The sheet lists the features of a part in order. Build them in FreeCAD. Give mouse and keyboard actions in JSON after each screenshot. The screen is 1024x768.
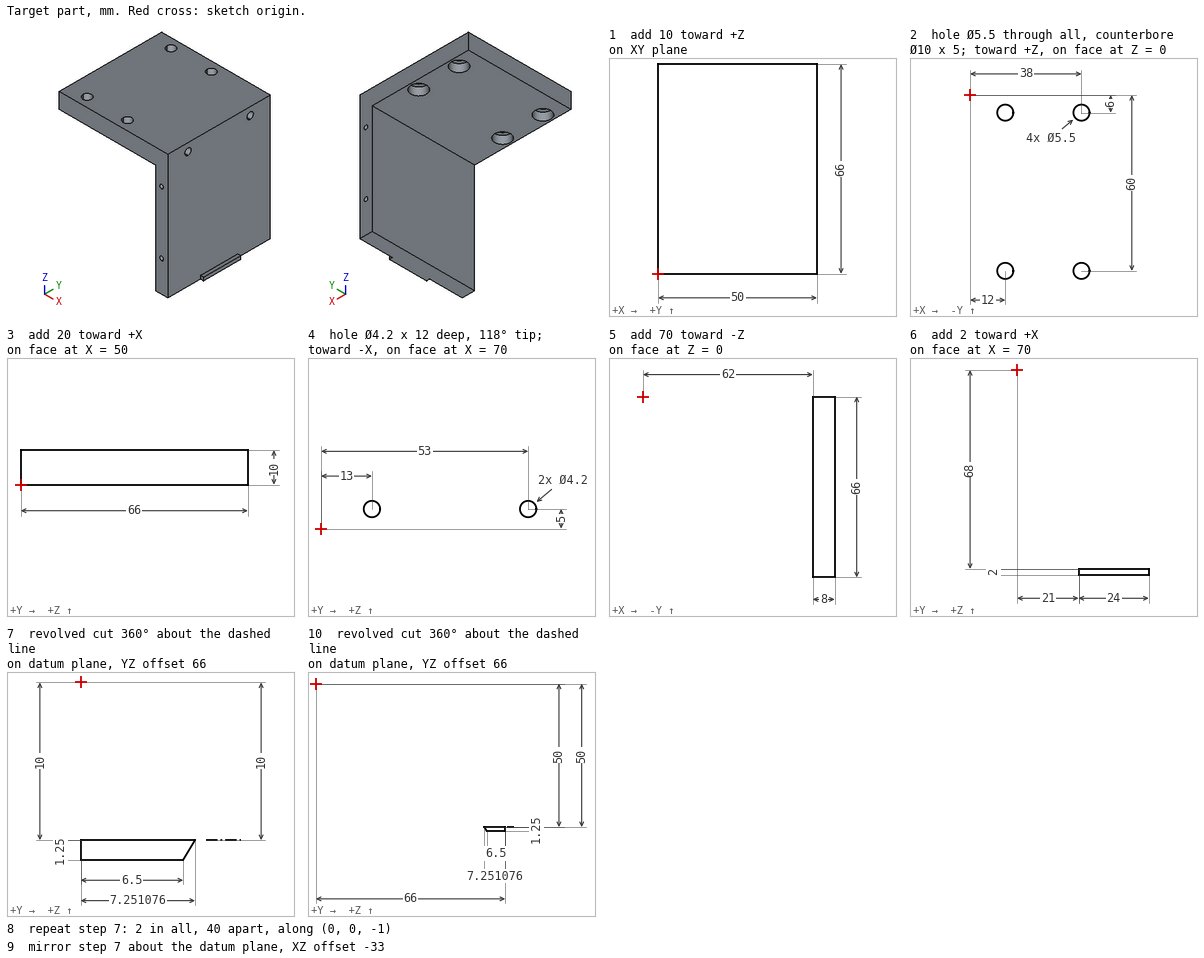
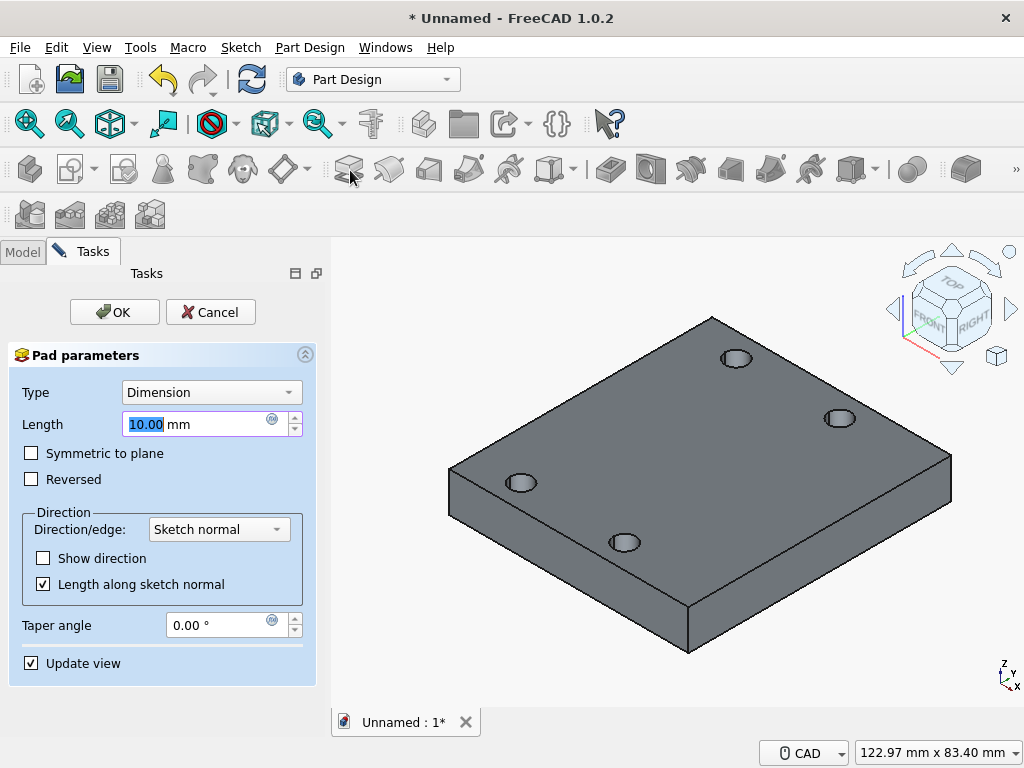
{"action": "type", "text": "20"}
{"action": "key", "text": "Tab"}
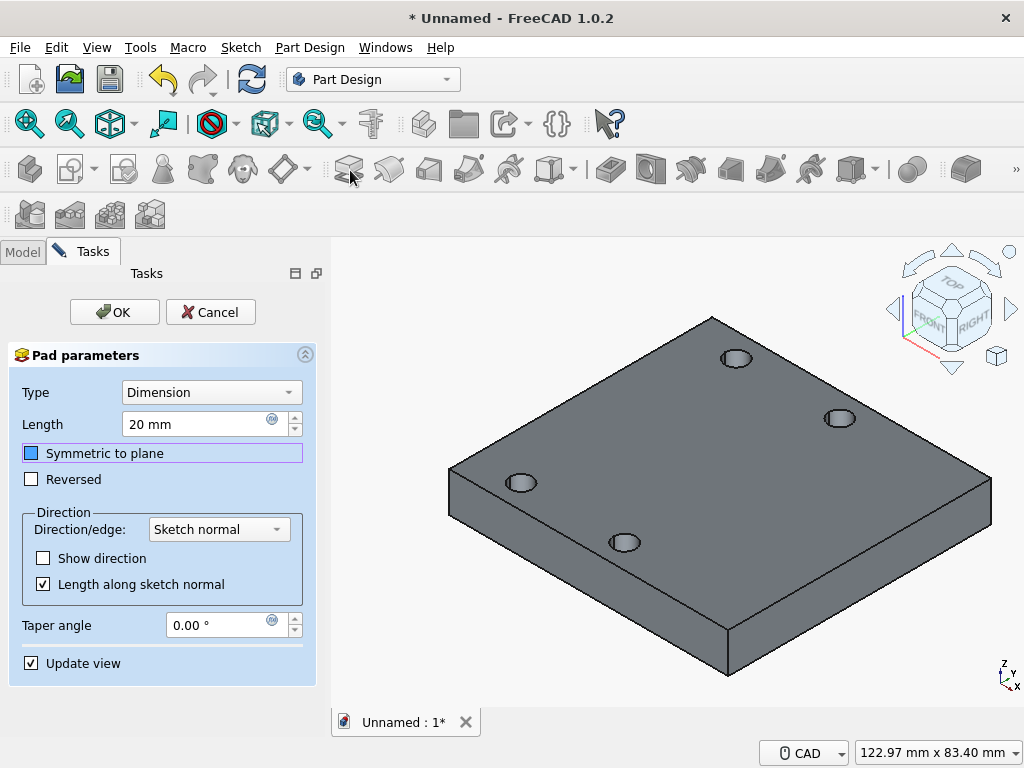
{"action": "left_click", "coordinate": [115, 312]}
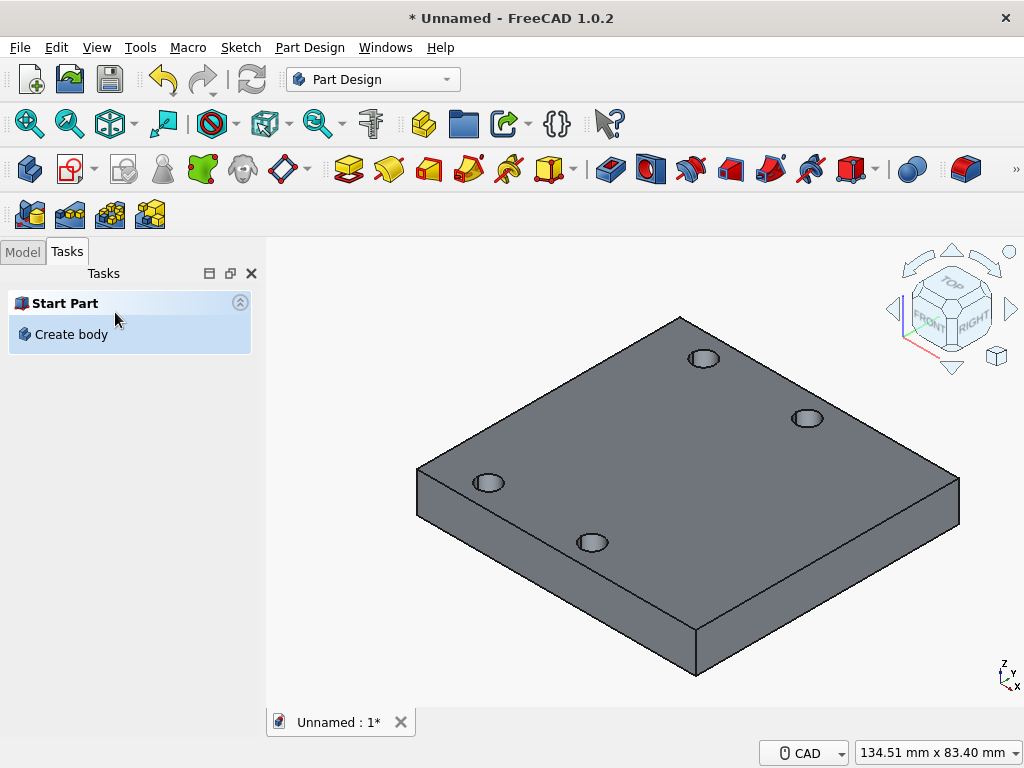
{"action": "left_click", "coordinate": [902, 533]}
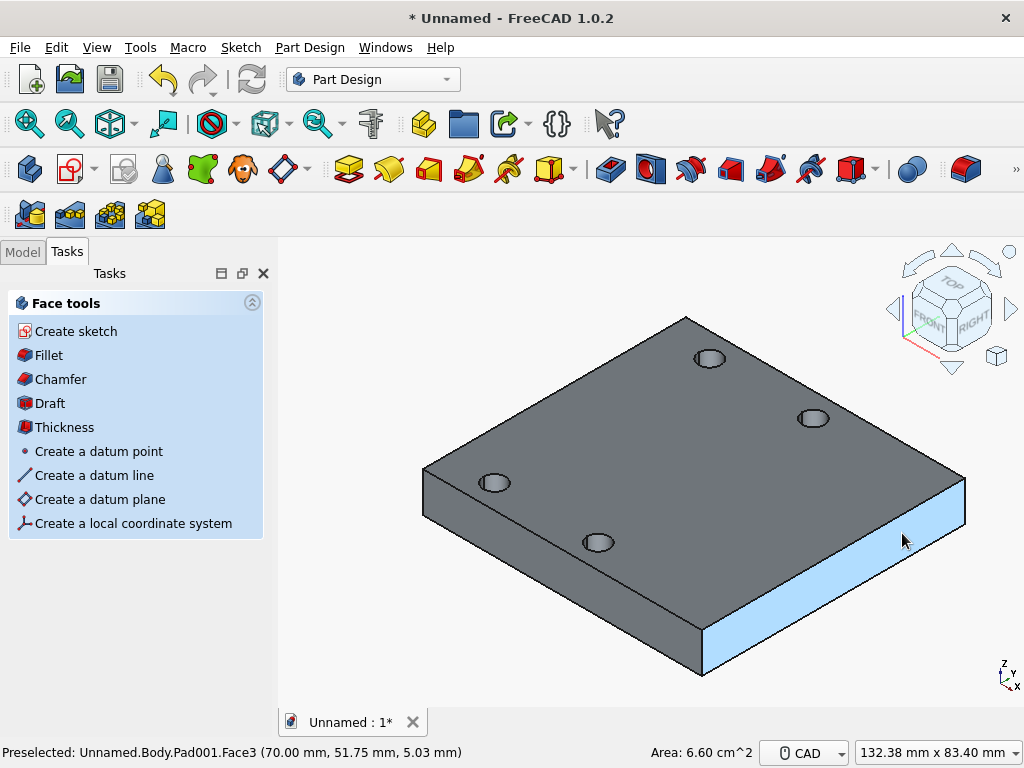
{"action": "left_click", "coordinate": [70, 170]}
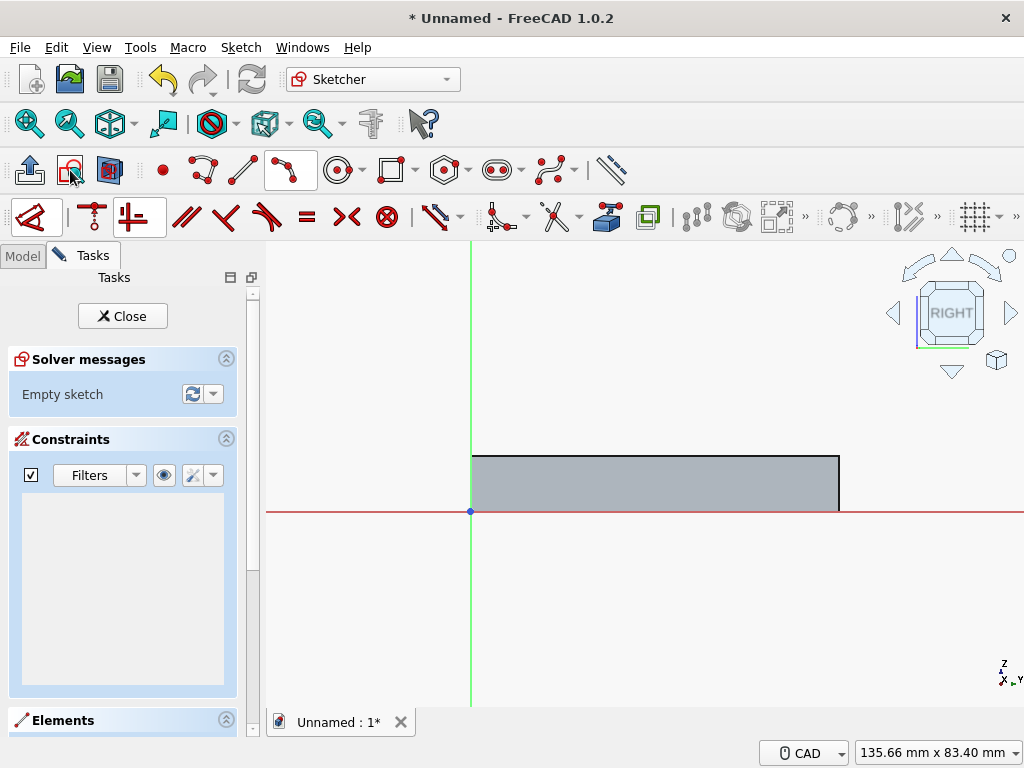
{"action": "key", "text": "g c"}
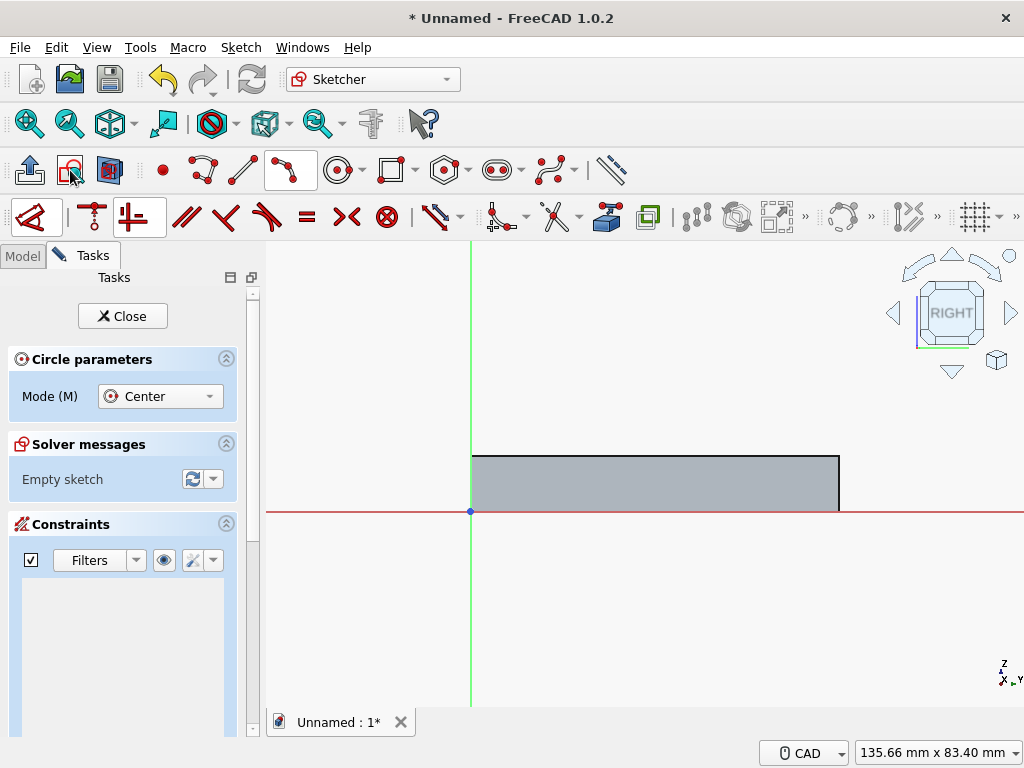
{"action": "scroll", "coordinate": [767, 484], "scroll_direction": "up", "scroll_amount": 4}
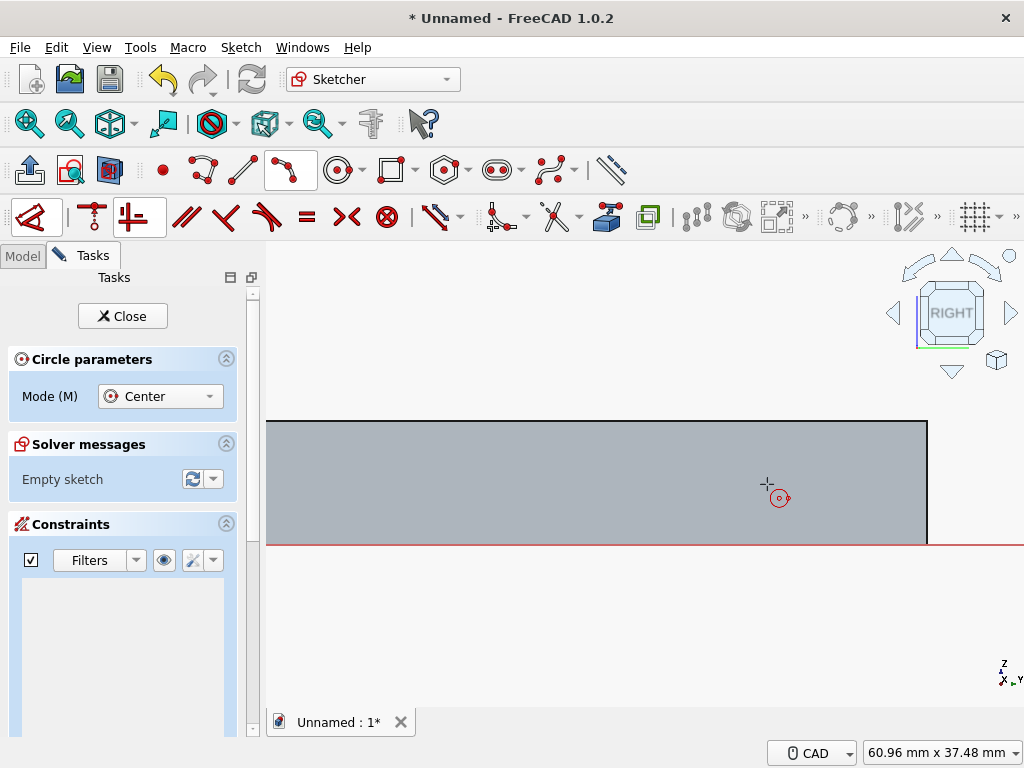
{"action": "left_click", "coordinate": [765, 483]}
{"action": "left_click", "coordinate": [784, 465]}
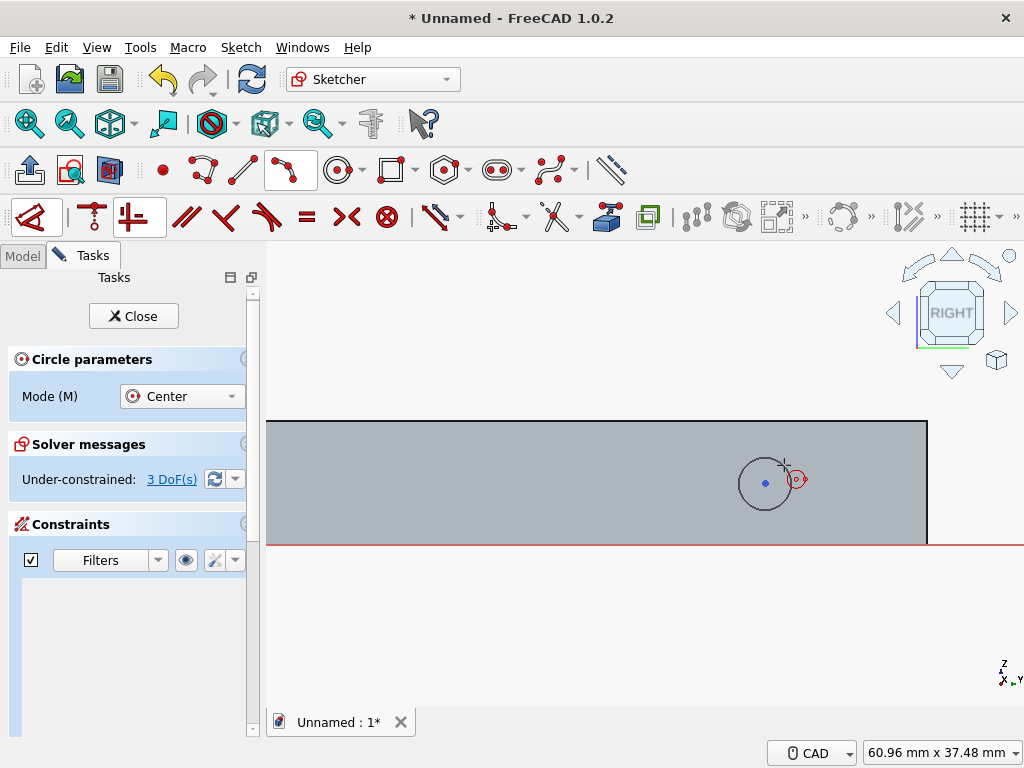
{"action": "scroll", "coordinate": [732, 441], "scroll_direction": "down", "scroll_amount": 3}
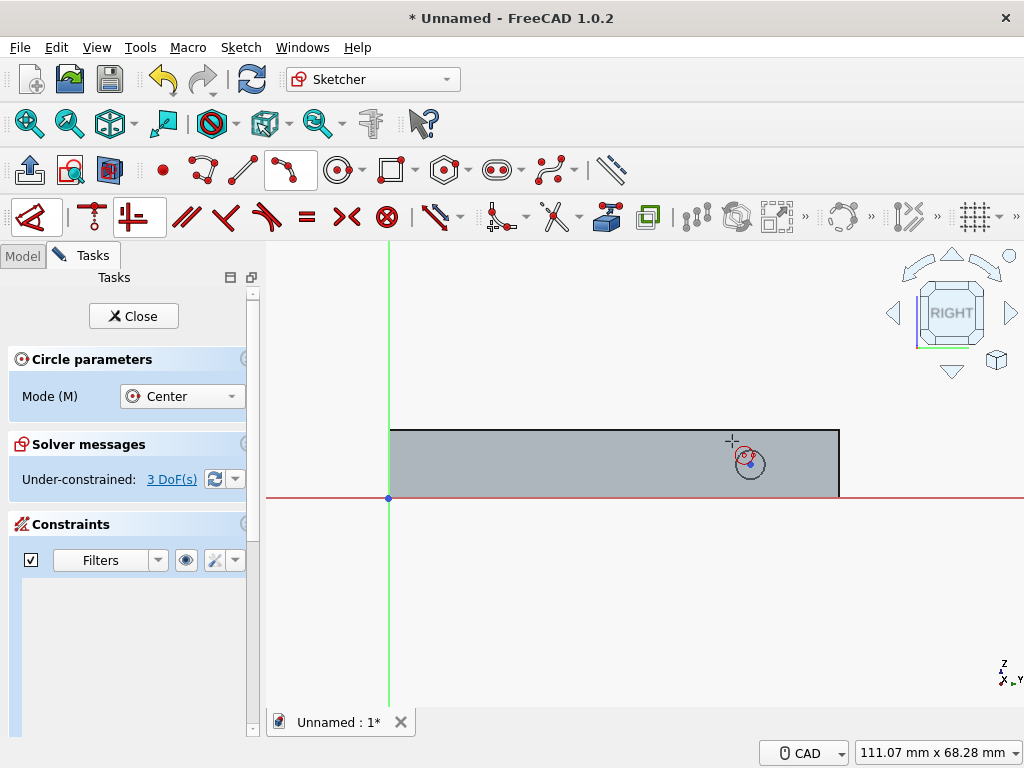
{"action": "scroll", "coordinate": [478, 464], "scroll_direction": "up", "scroll_amount": 3}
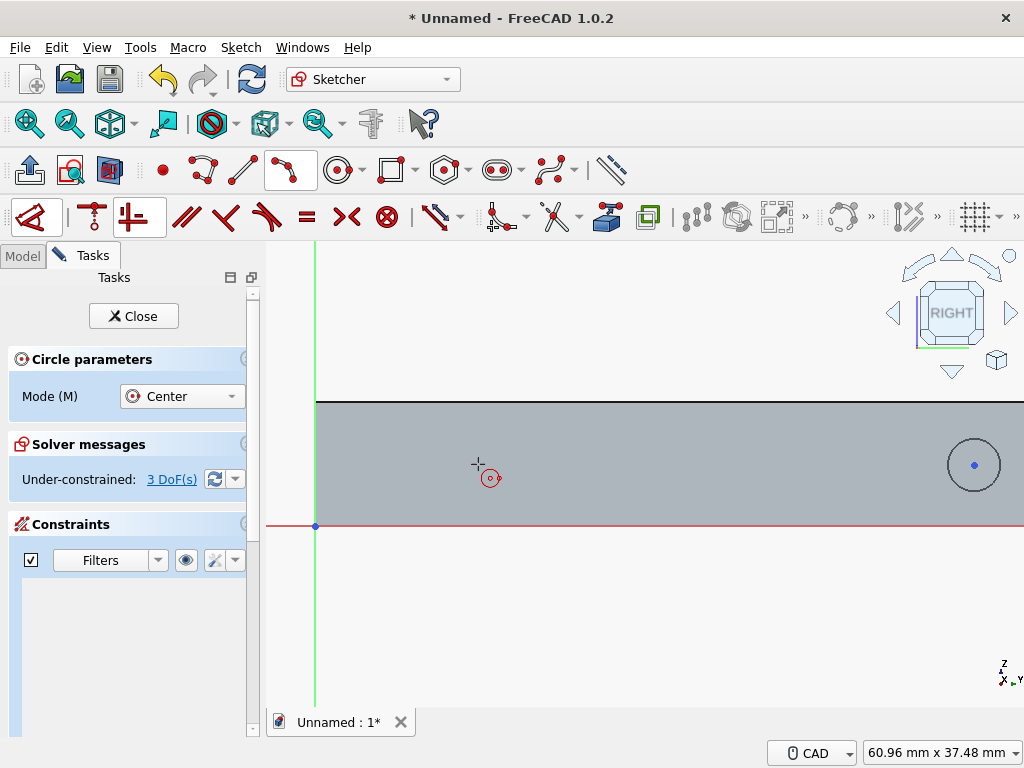
{"action": "left_click", "coordinate": [477, 464]}
{"action": "left_click", "coordinate": [496, 446]}
{"action": "key", "text": "Escape"}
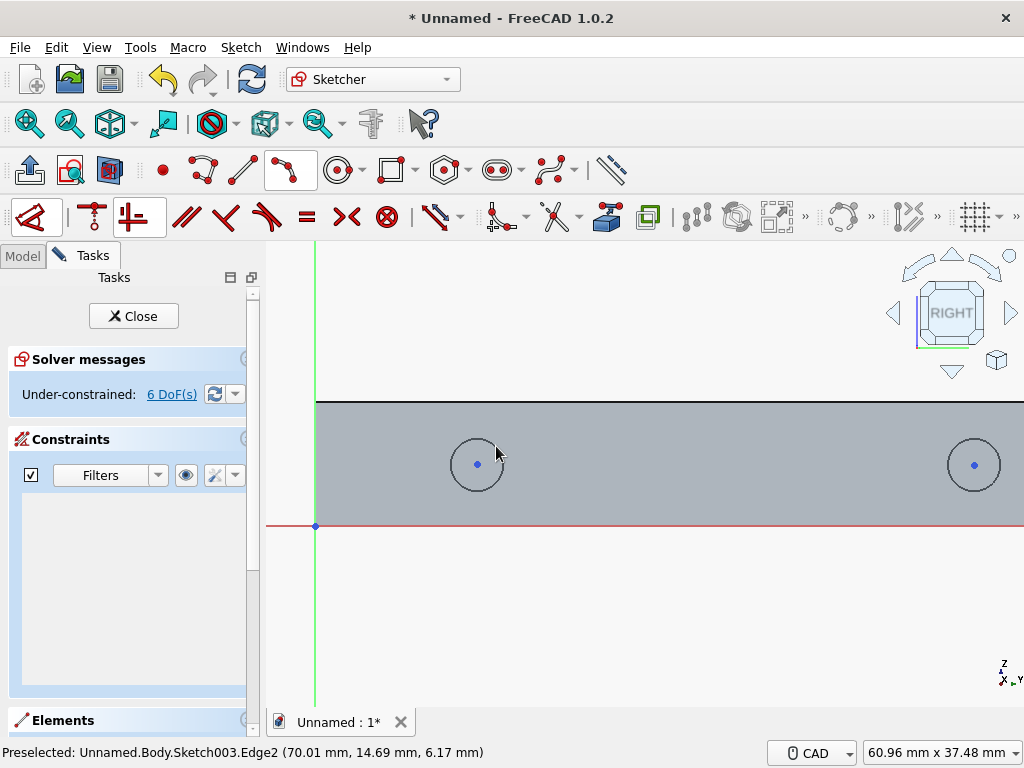
{"action": "scroll", "coordinate": [477, 464], "scroll_direction": "down", "scroll_amount": 3}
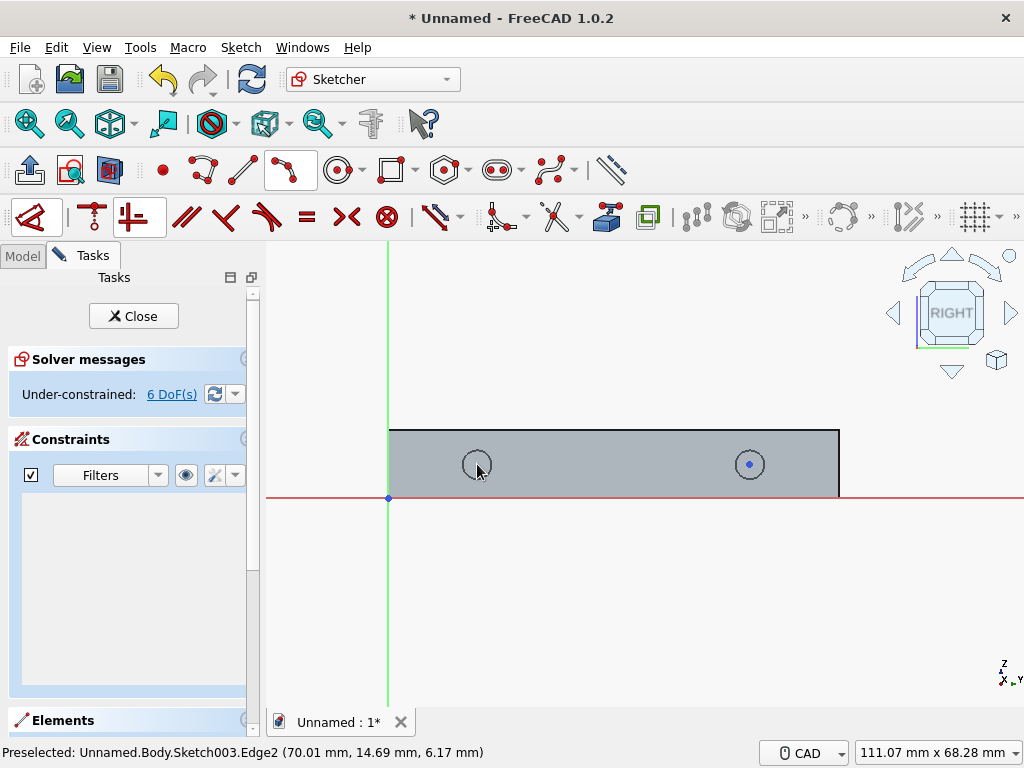
{"action": "left_click", "coordinate": [760, 455]}